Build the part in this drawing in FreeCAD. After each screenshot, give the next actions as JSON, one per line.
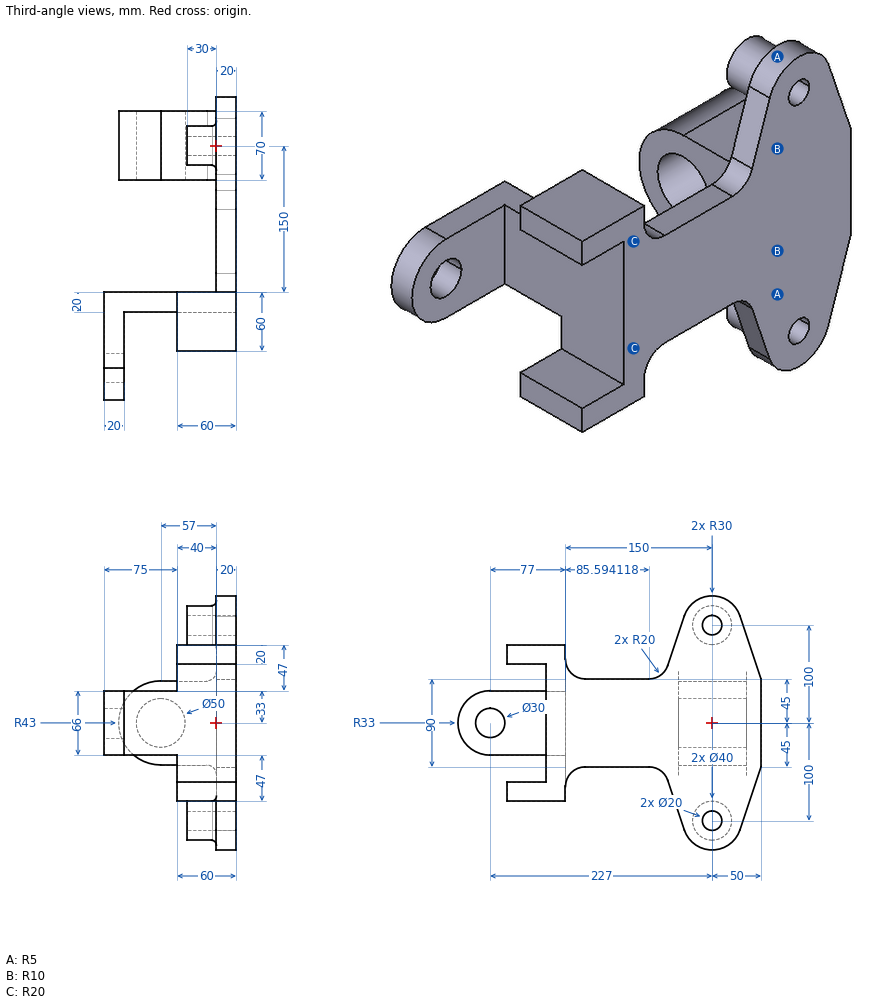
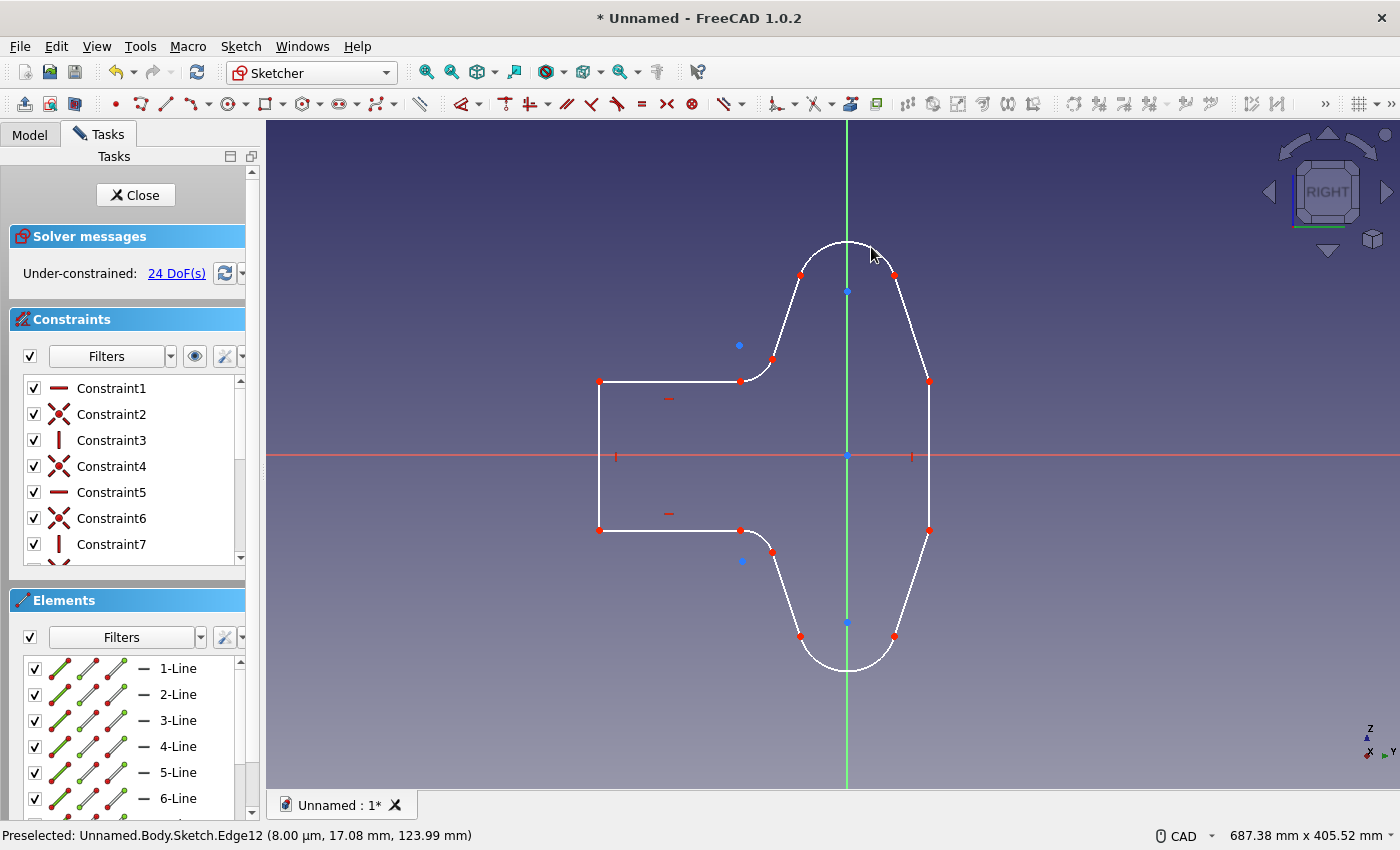
{"action": "left_click", "coordinate": [792, 301]}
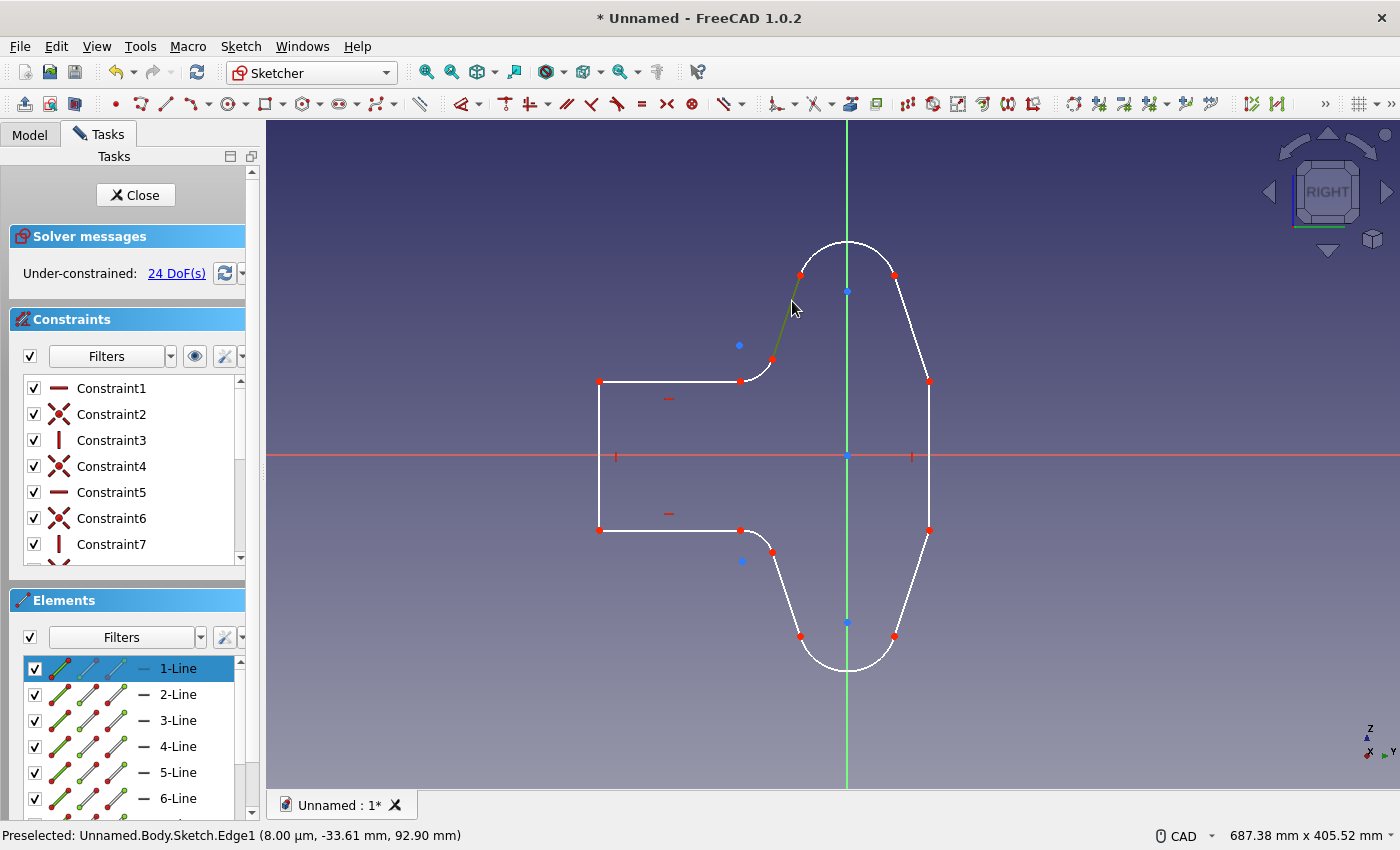
{"action": "left_click", "coordinate": [752, 379]}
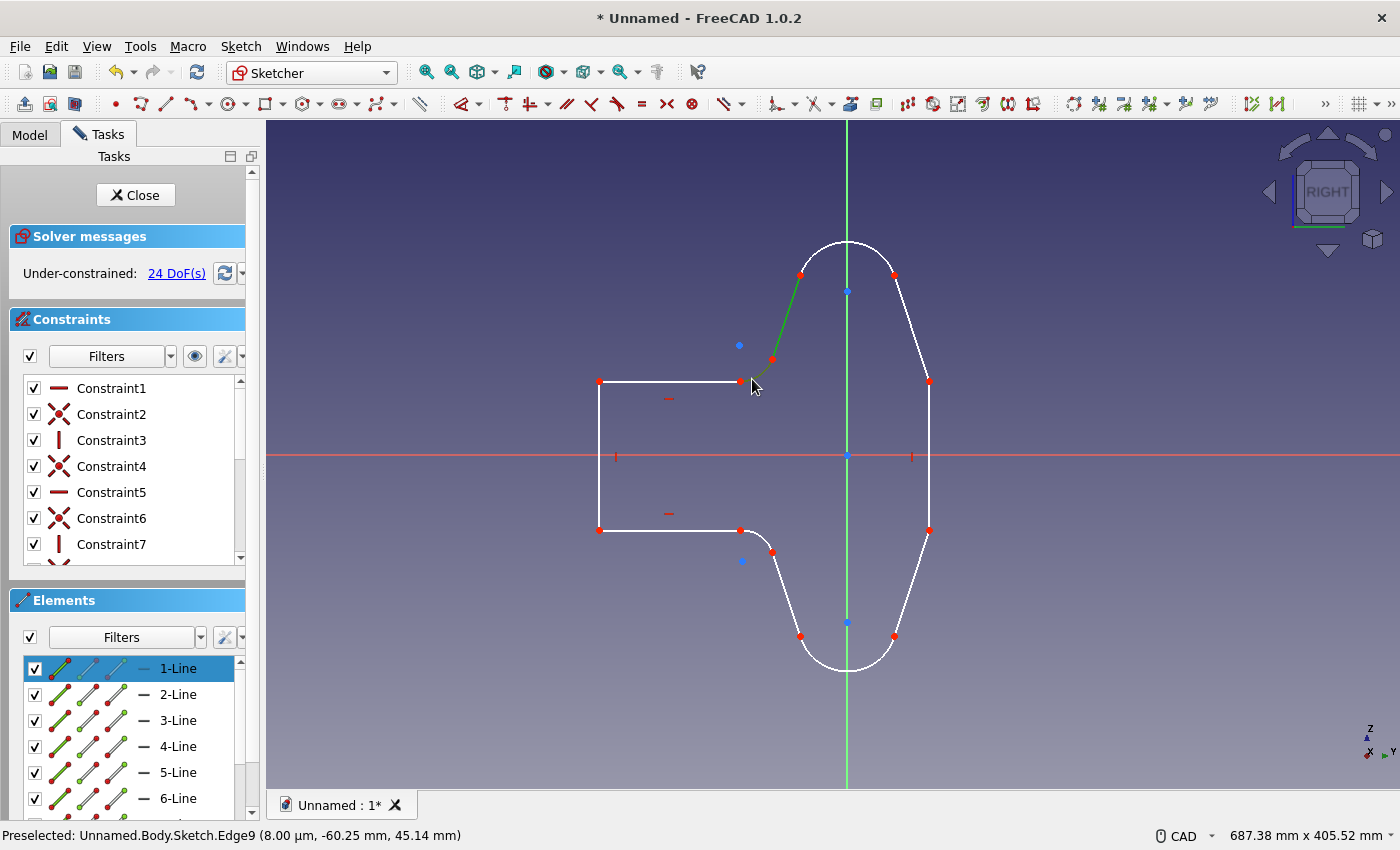
{"action": "left_click", "coordinate": [617, 104]}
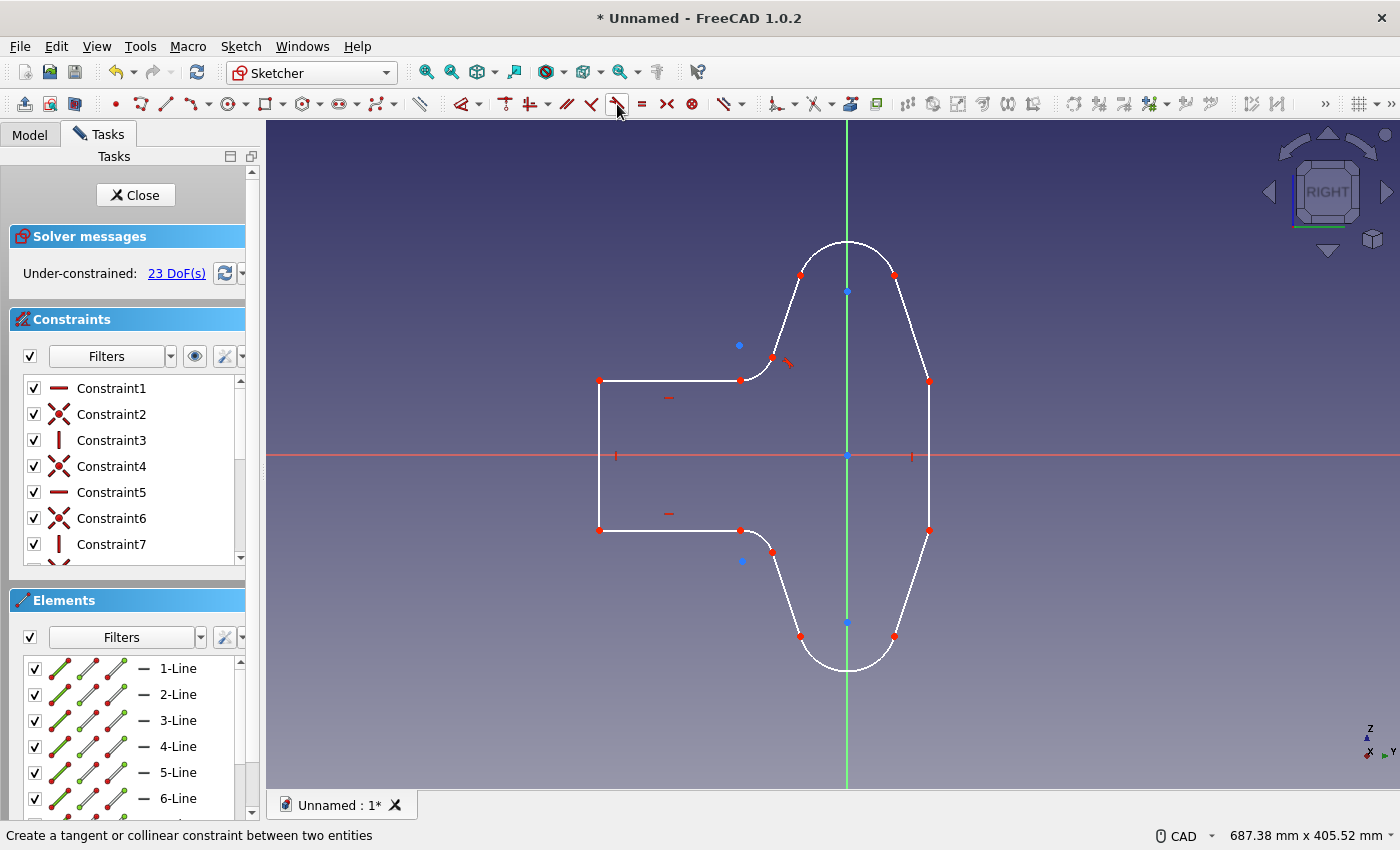
{"action": "left_click", "coordinate": [792, 300]}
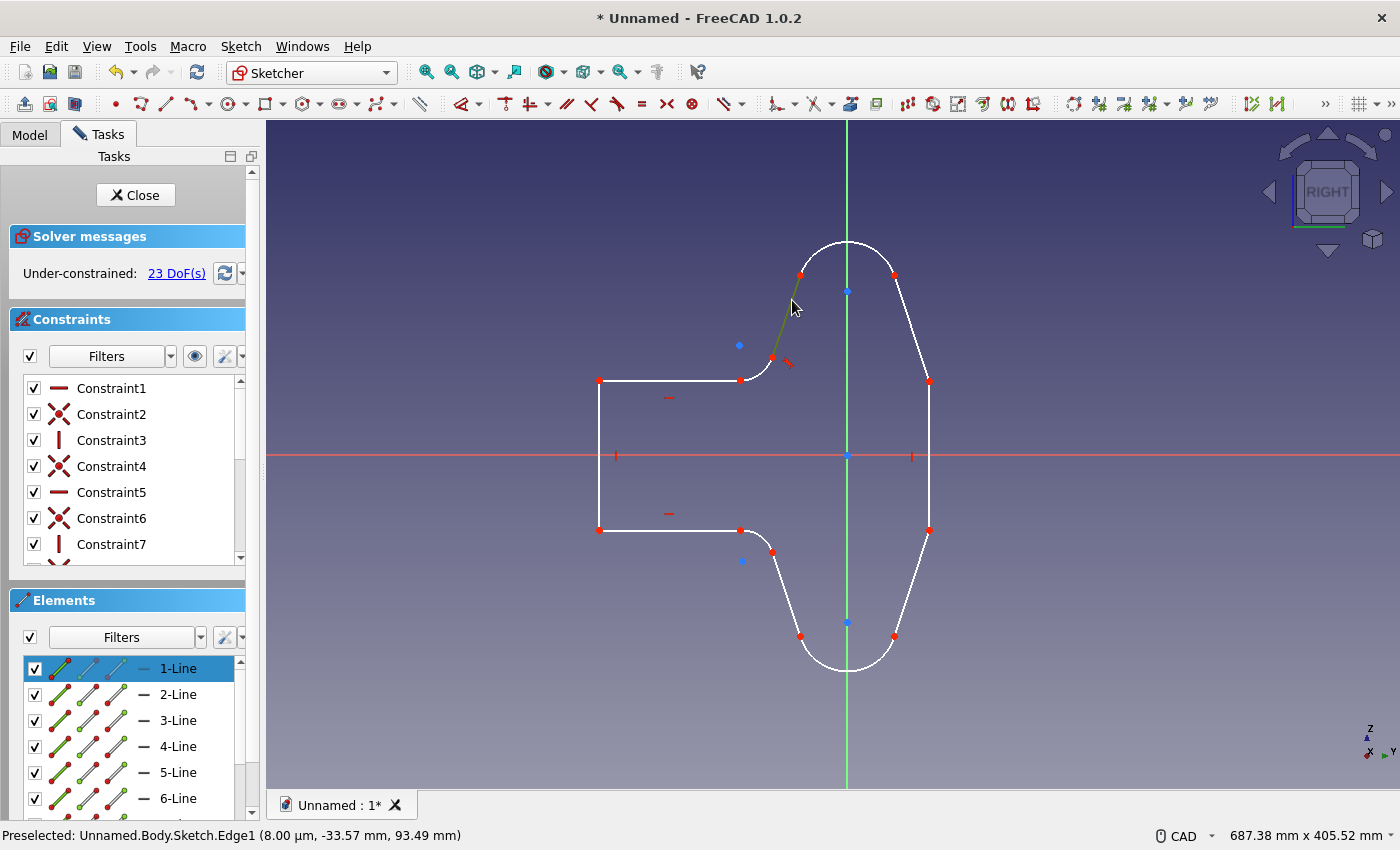
{"action": "left_click", "coordinate": [871, 248]}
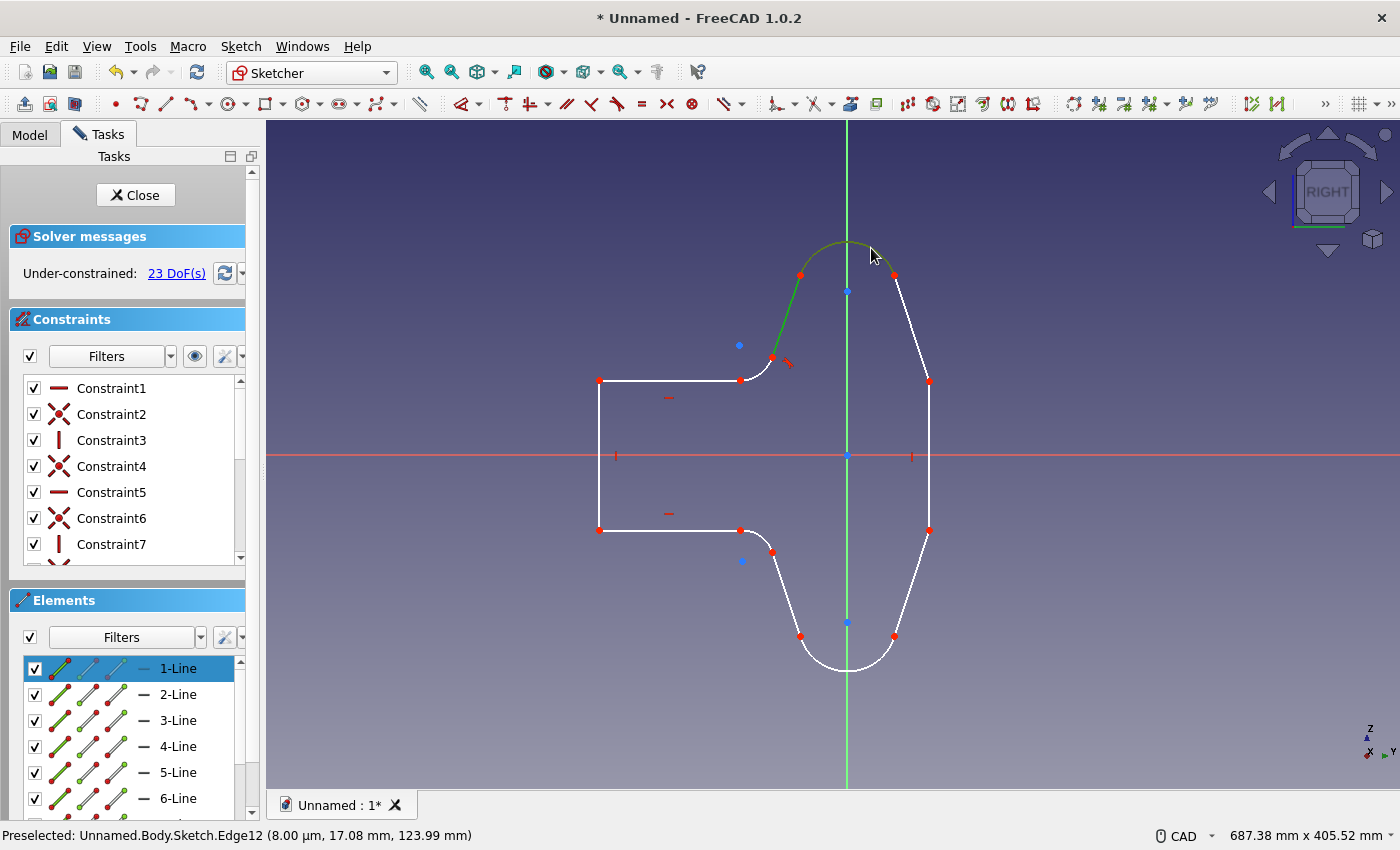
{"action": "left_click", "coordinate": [617, 104]}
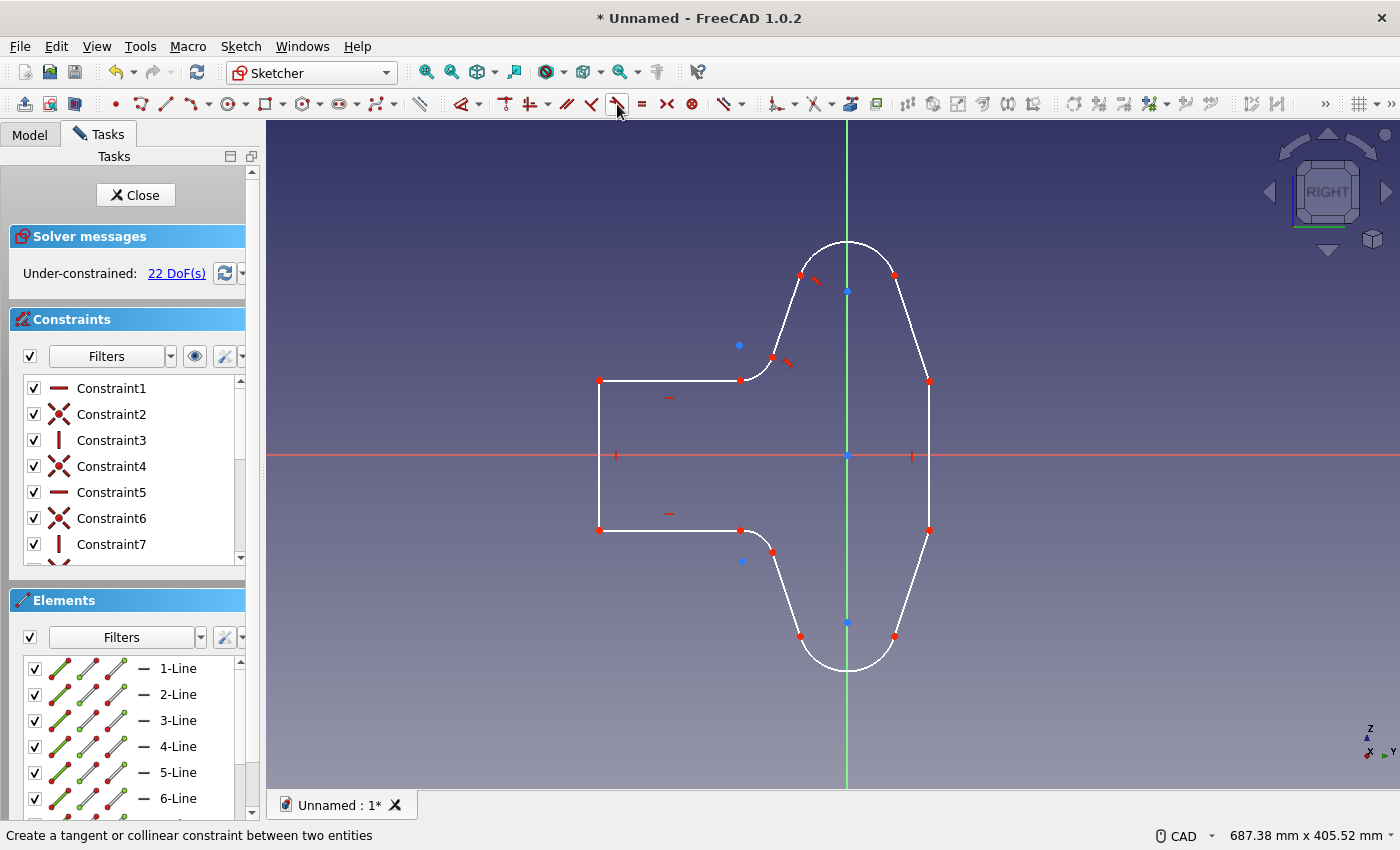
{"action": "left_click", "coordinate": [698, 381]}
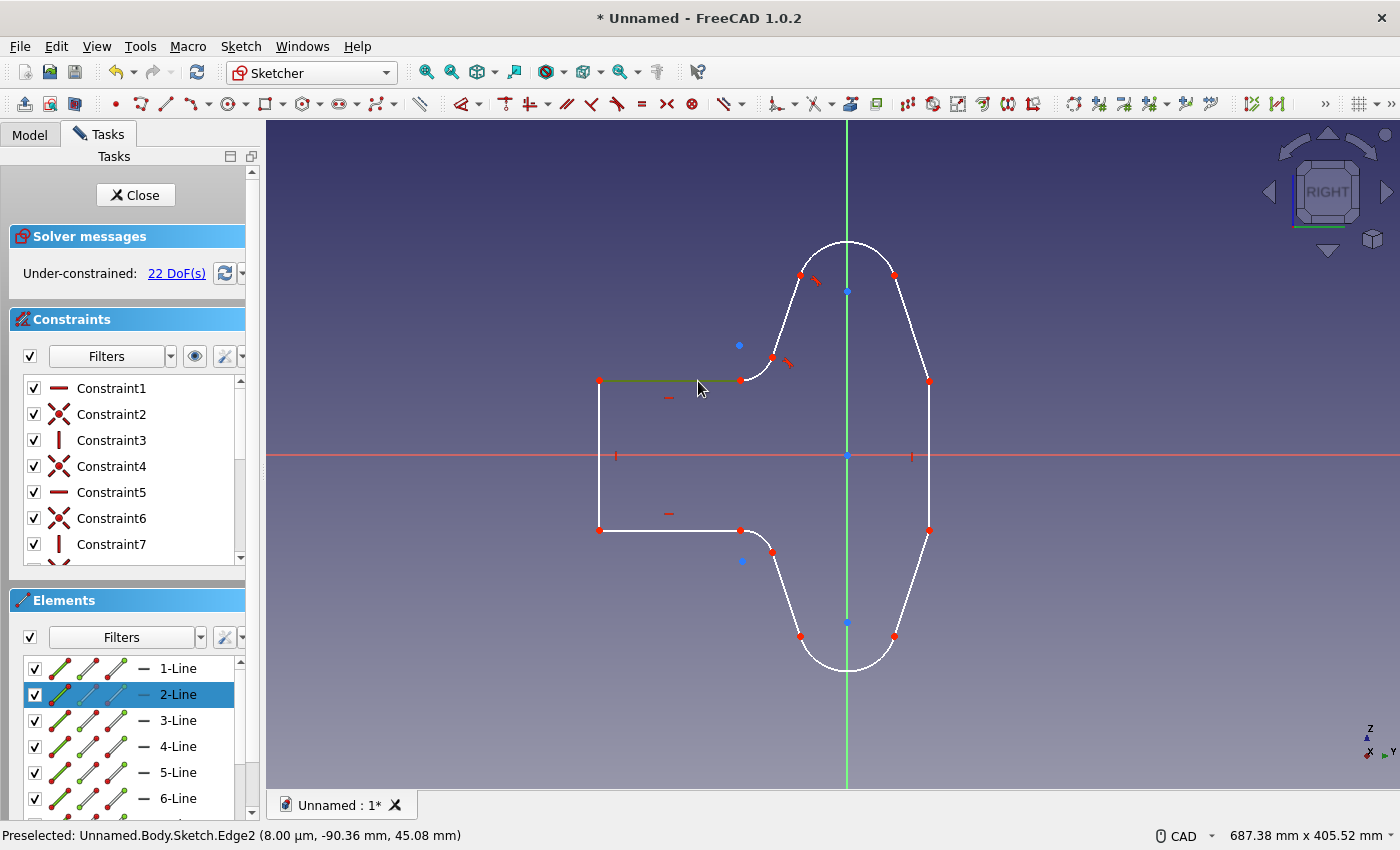
{"action": "left_click", "coordinate": [753, 378]}